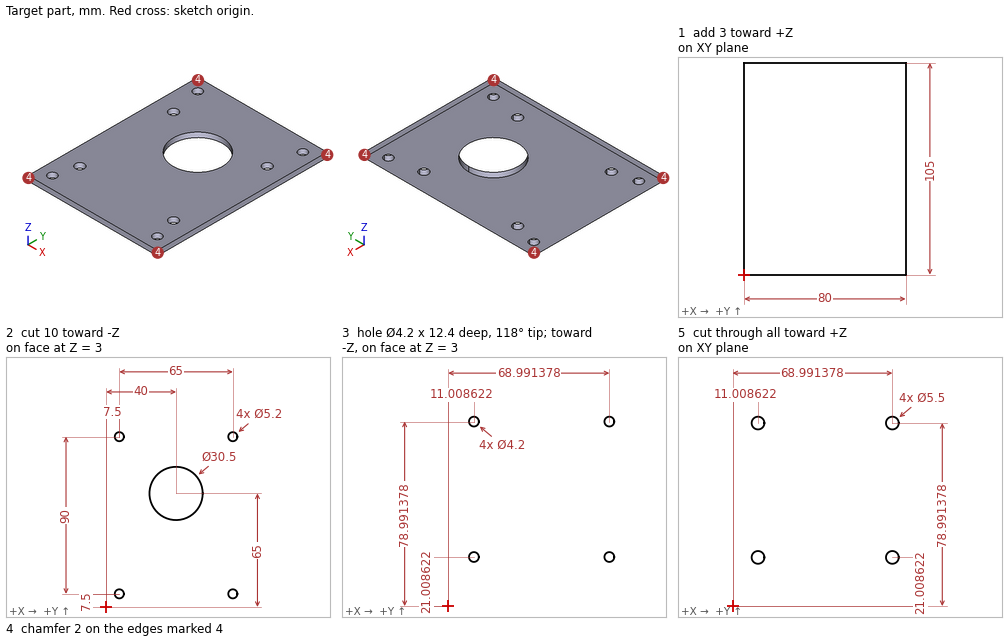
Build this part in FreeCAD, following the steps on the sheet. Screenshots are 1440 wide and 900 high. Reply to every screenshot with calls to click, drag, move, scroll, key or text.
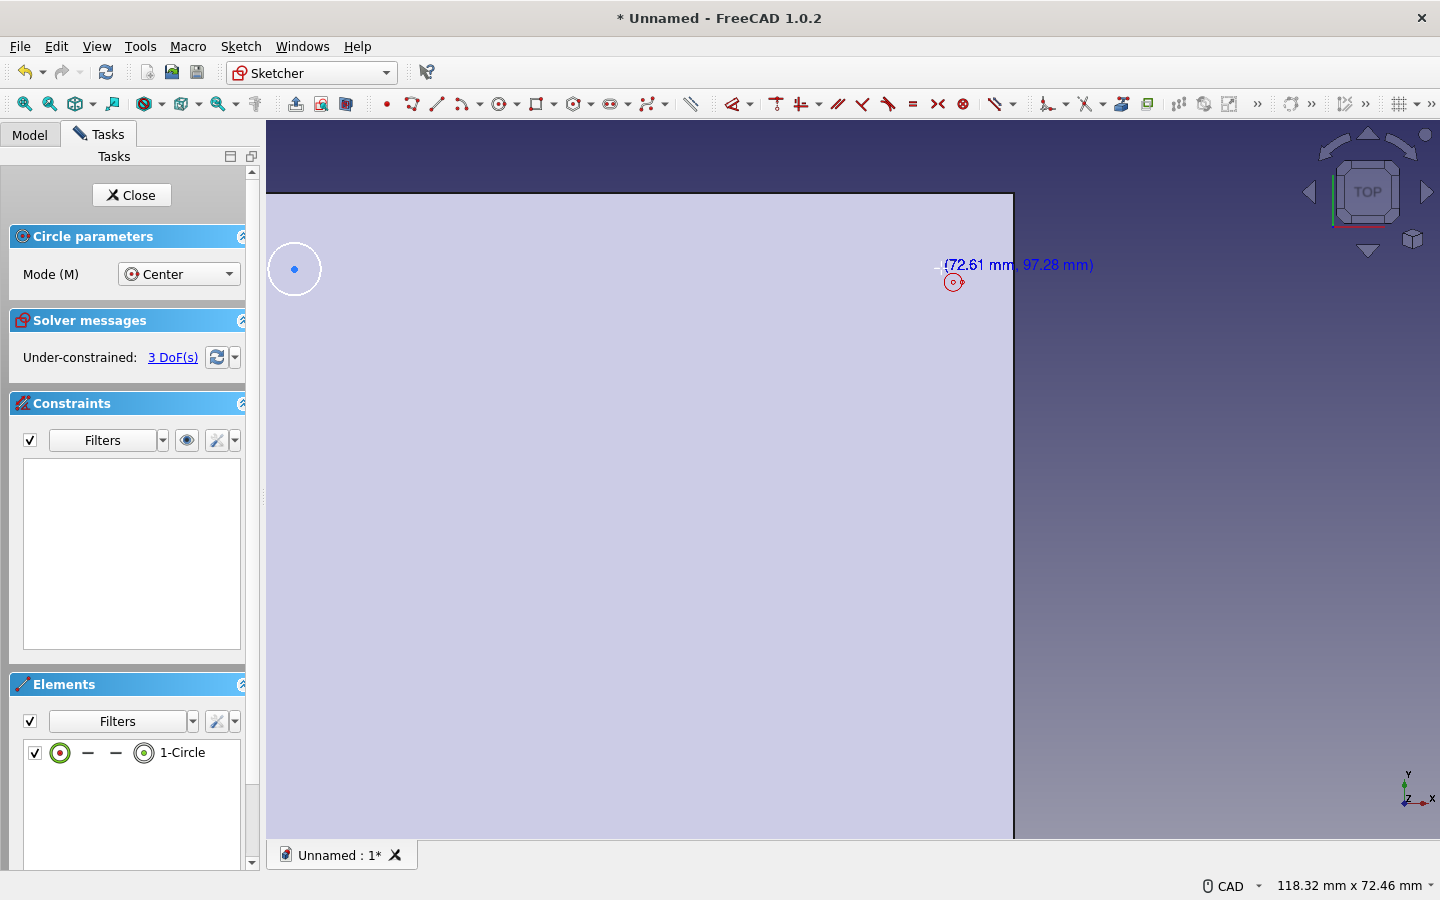
click(939, 268)
click(957, 250)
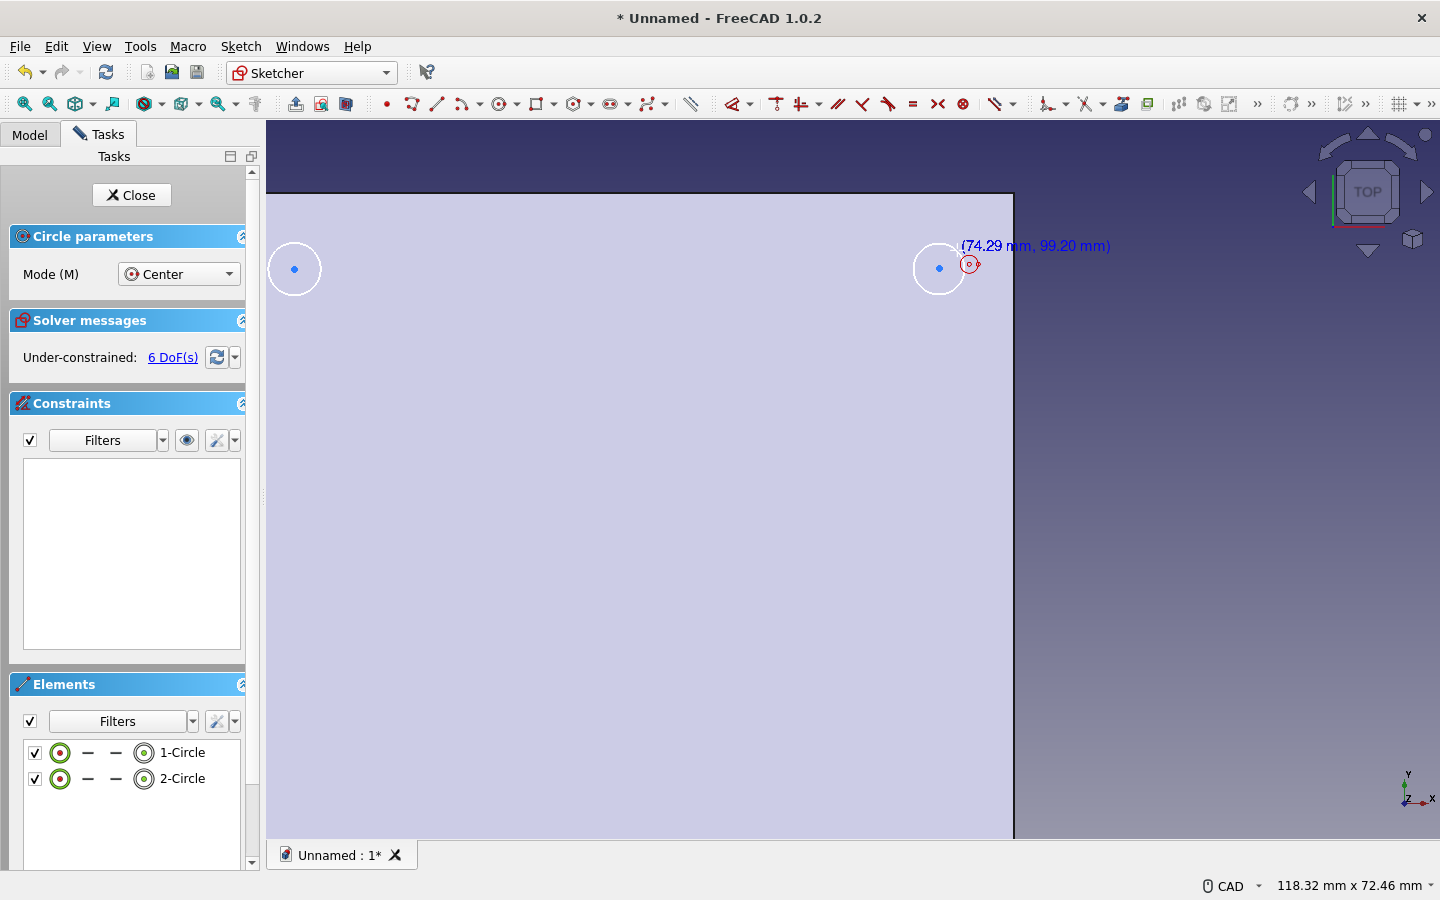
scroll(941, 268, down, 4)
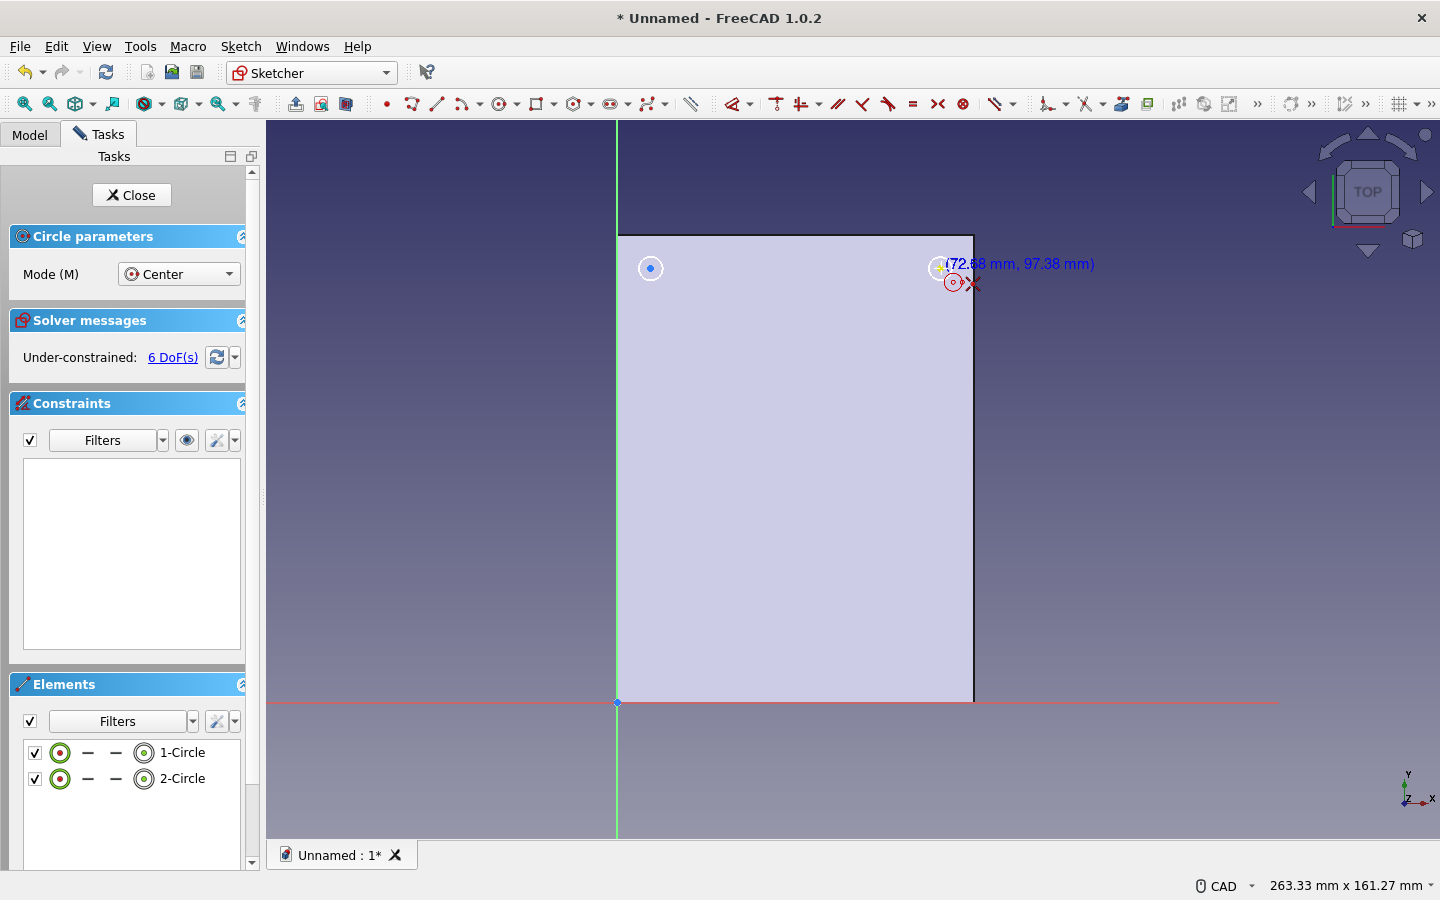
scroll(651, 669, up, 4)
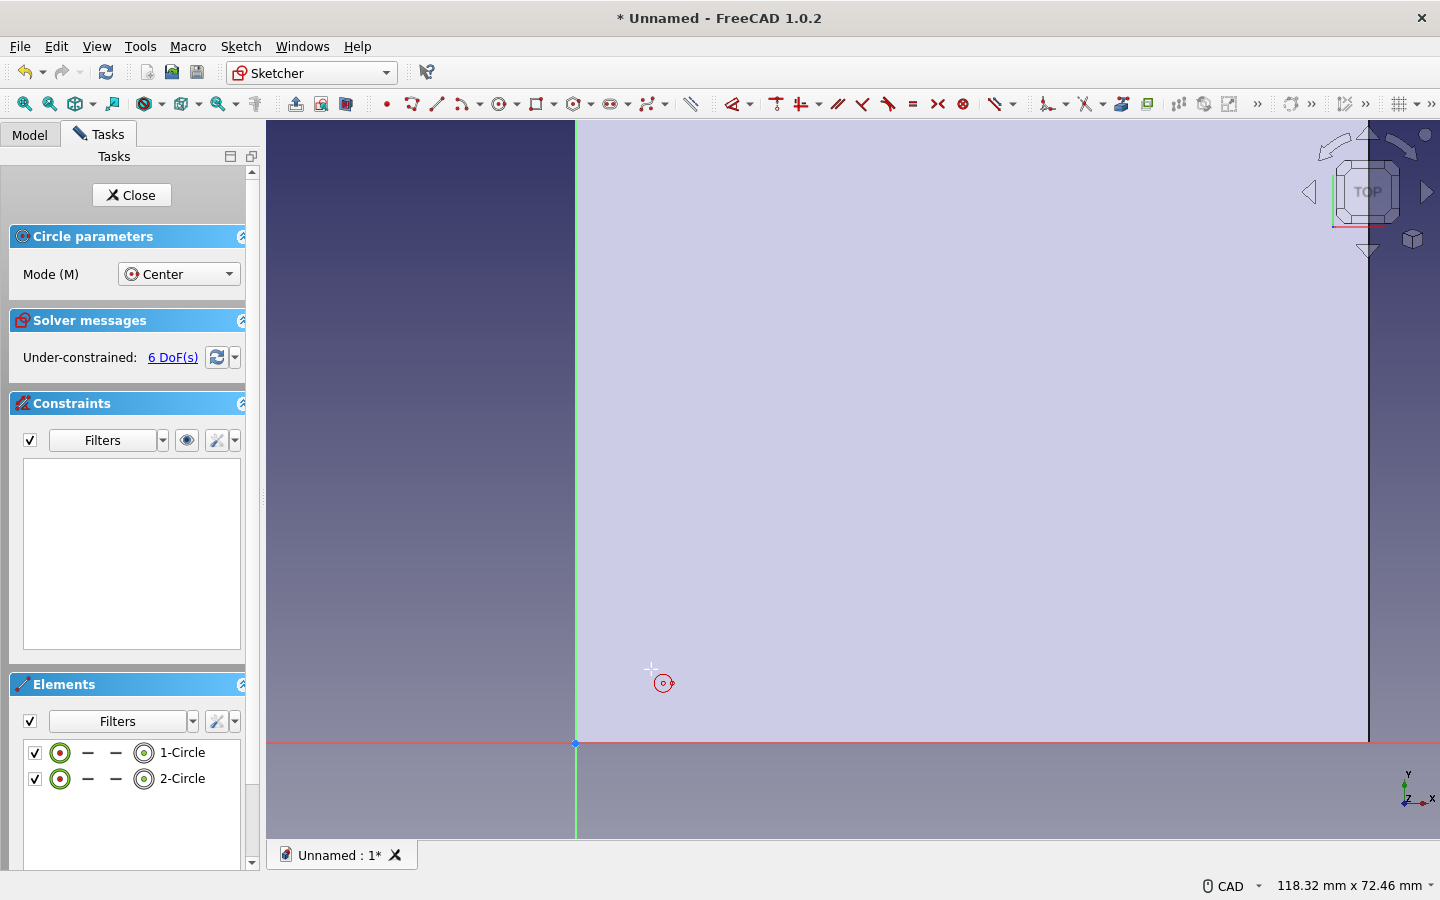
click(650, 669)
click(668, 650)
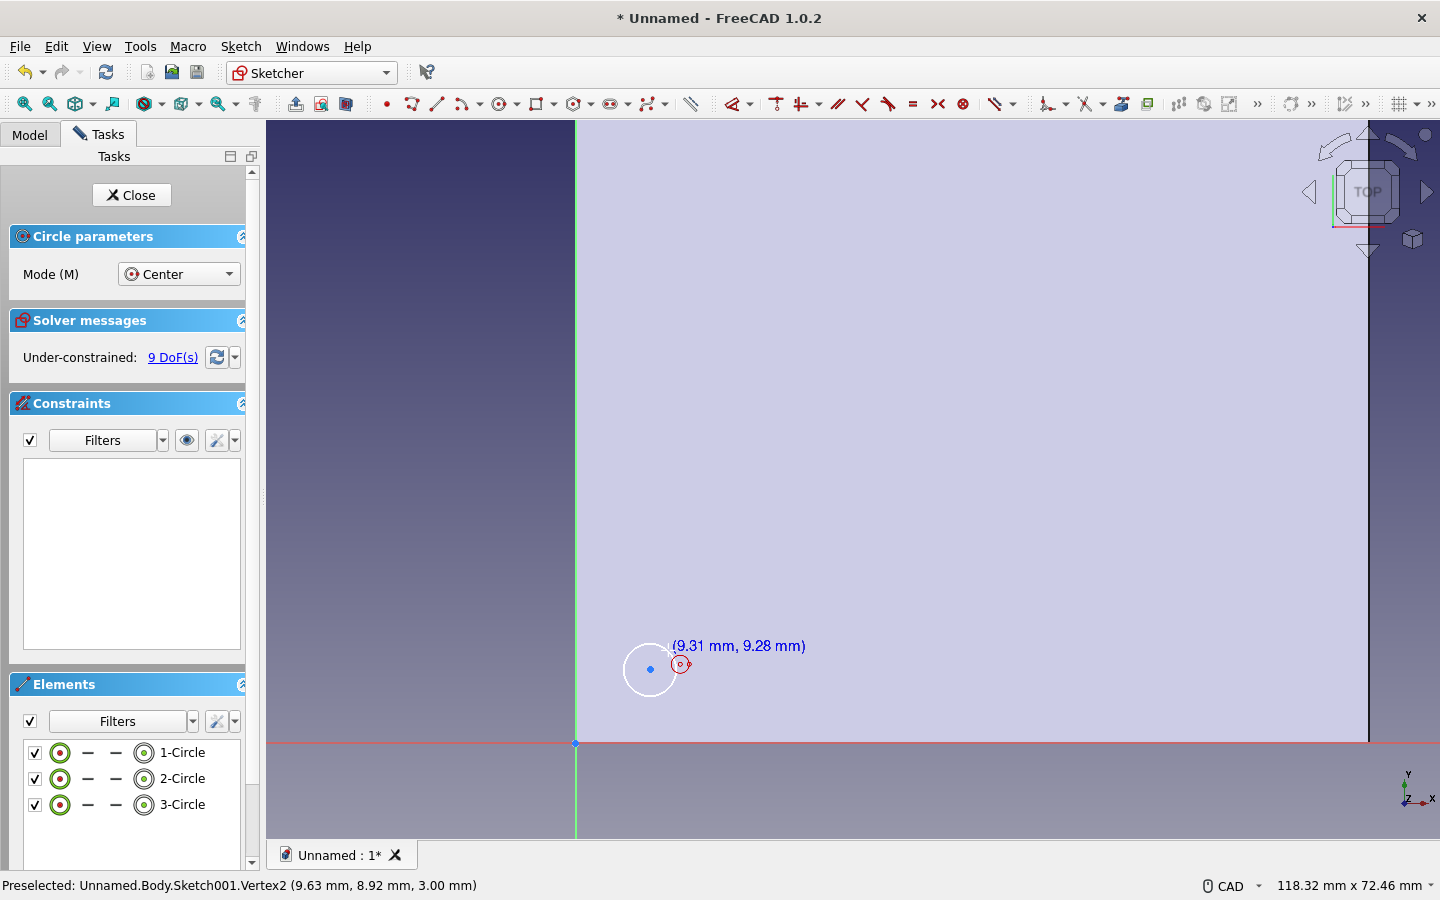
scroll(651, 670, down, 4)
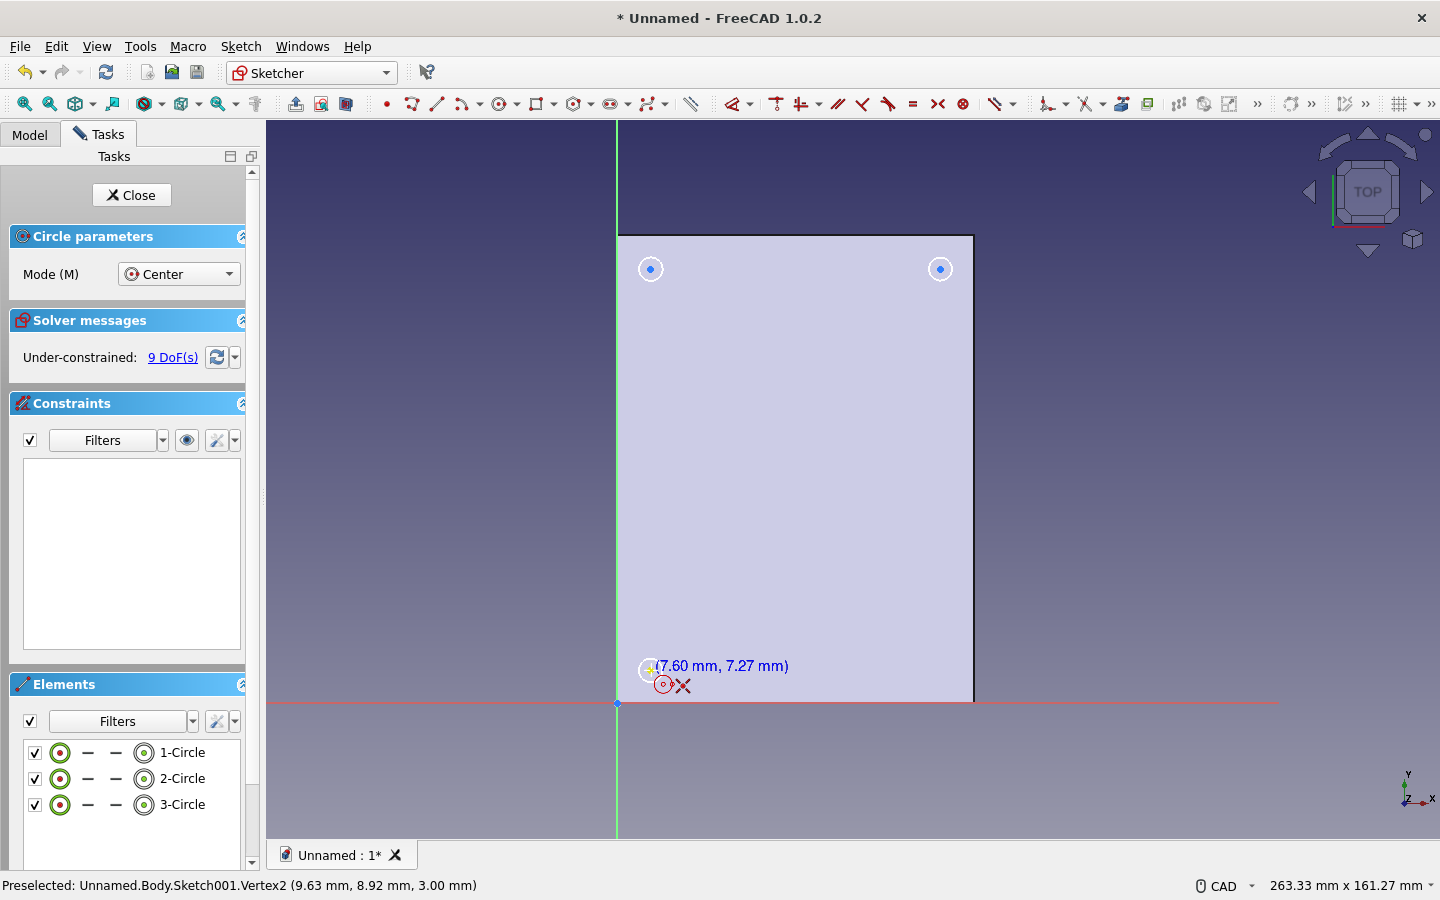
scroll(941, 670, up, 4)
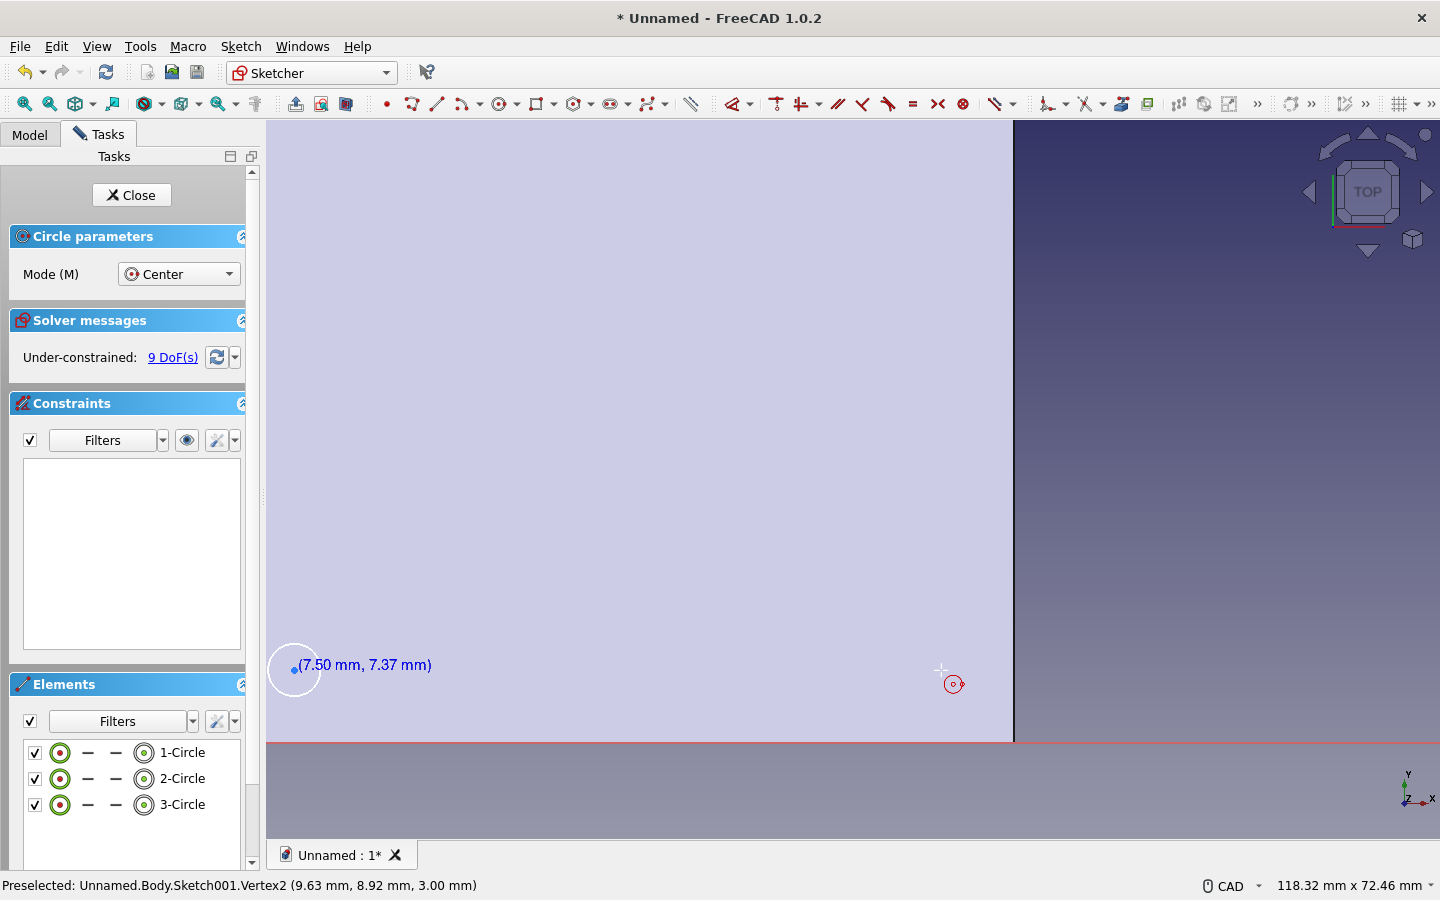
click(939, 669)
click(957, 650)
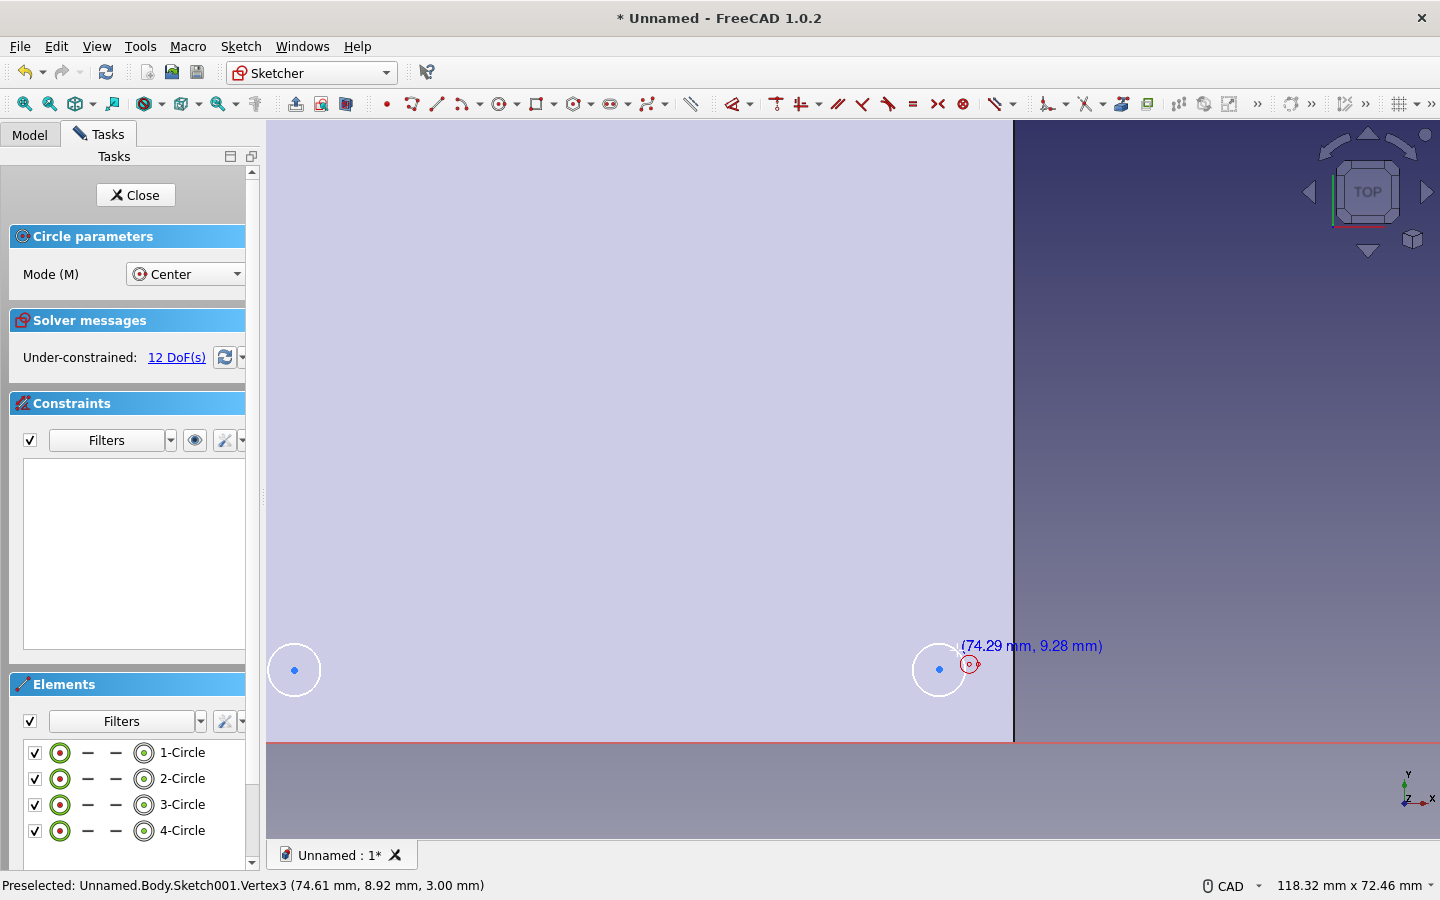
scroll(941, 670, down, 4)